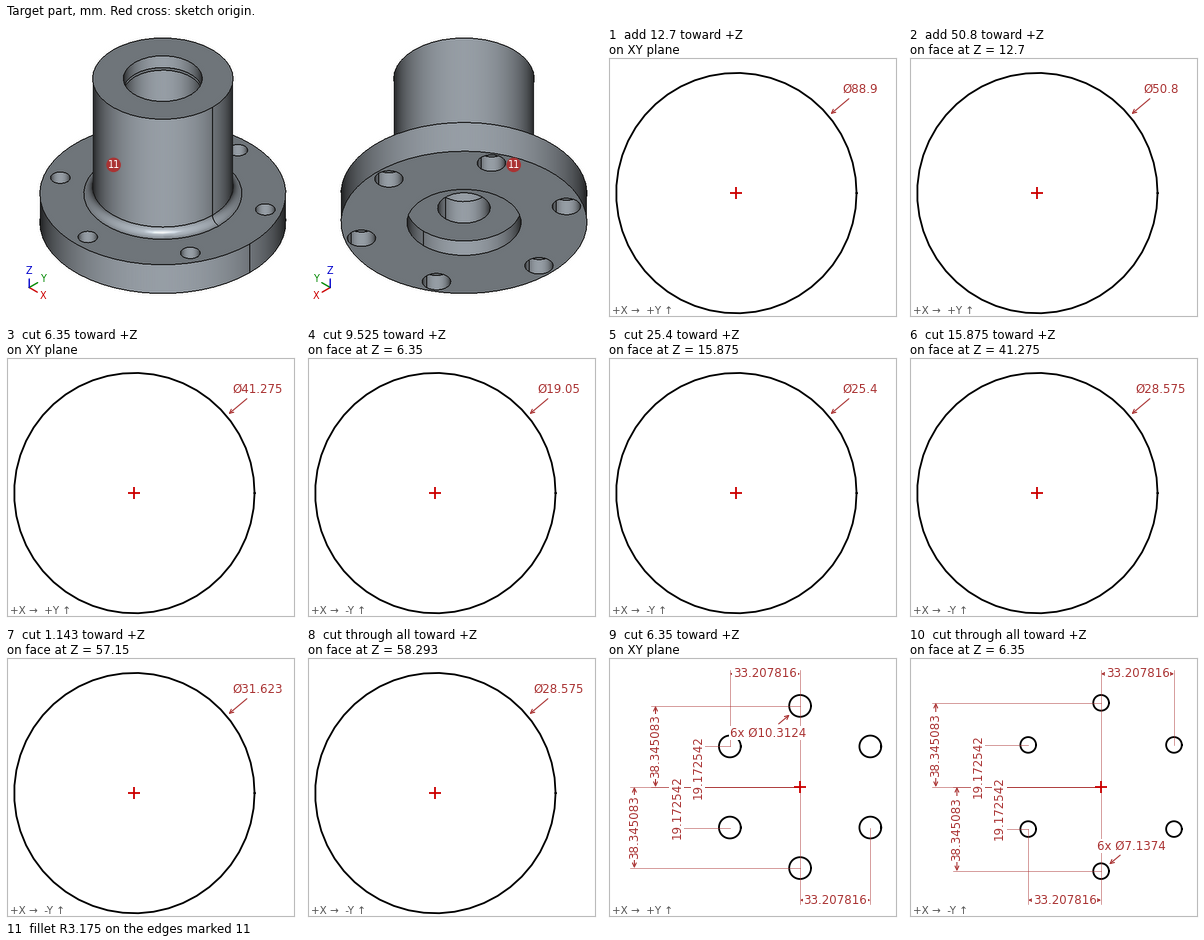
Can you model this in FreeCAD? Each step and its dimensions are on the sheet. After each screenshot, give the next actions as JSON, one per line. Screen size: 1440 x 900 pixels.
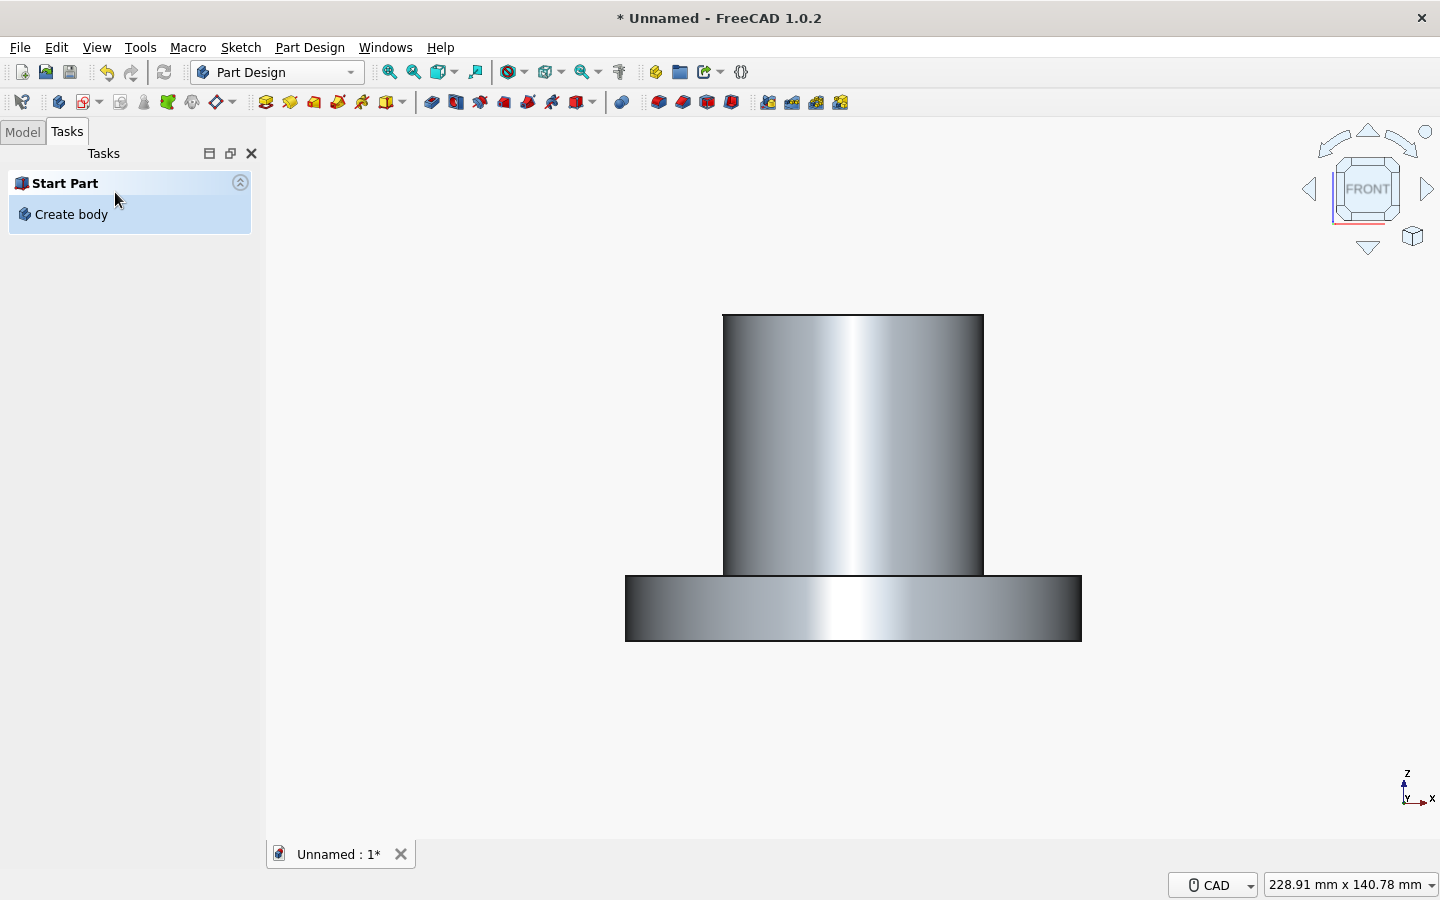
{"action": "key", "text": "3"}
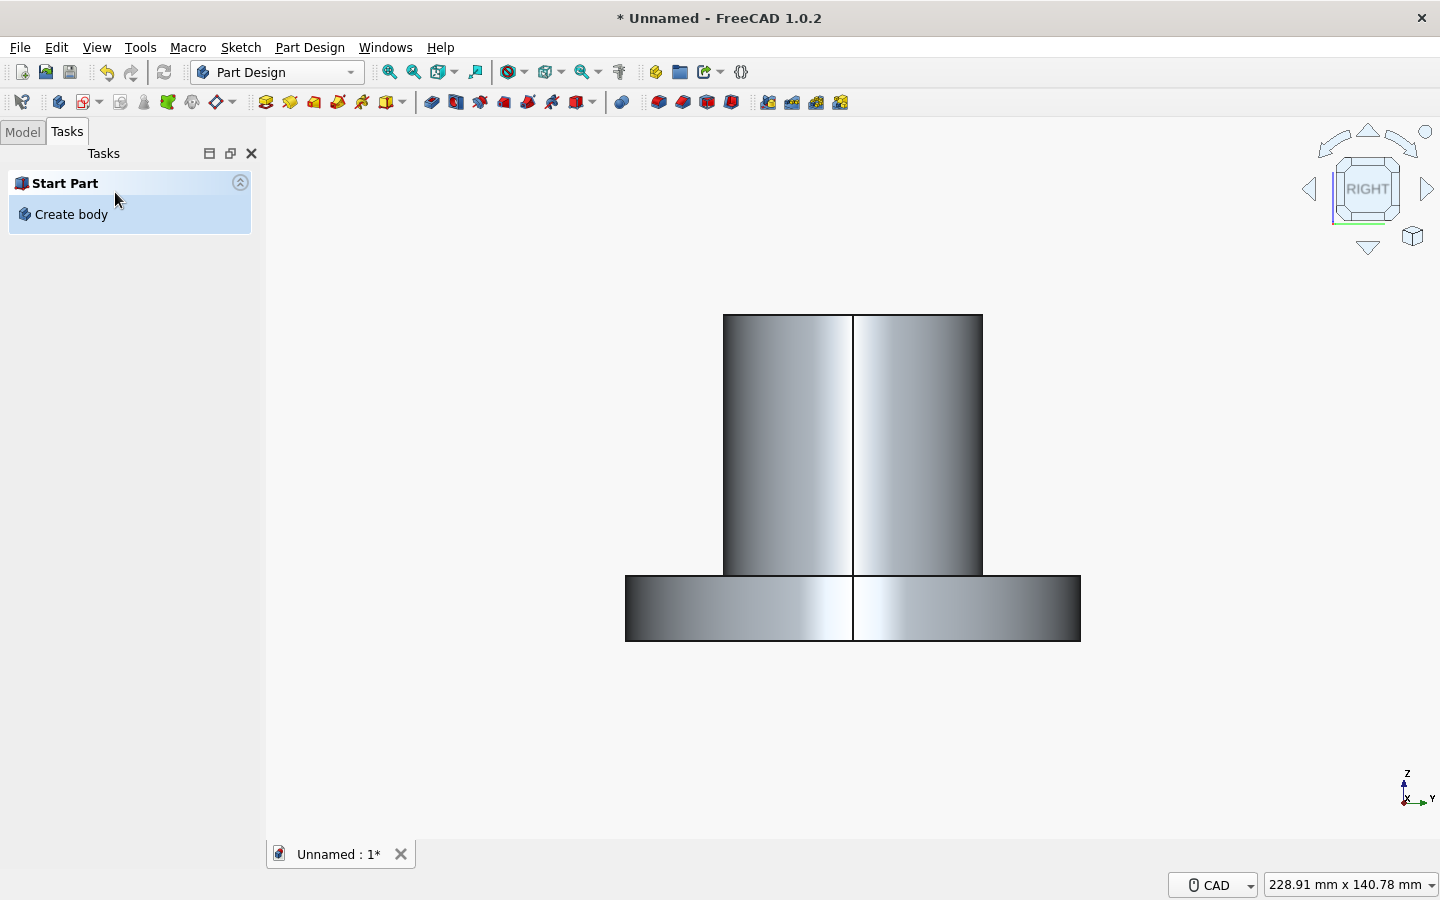
{"action": "key", "text": "5"}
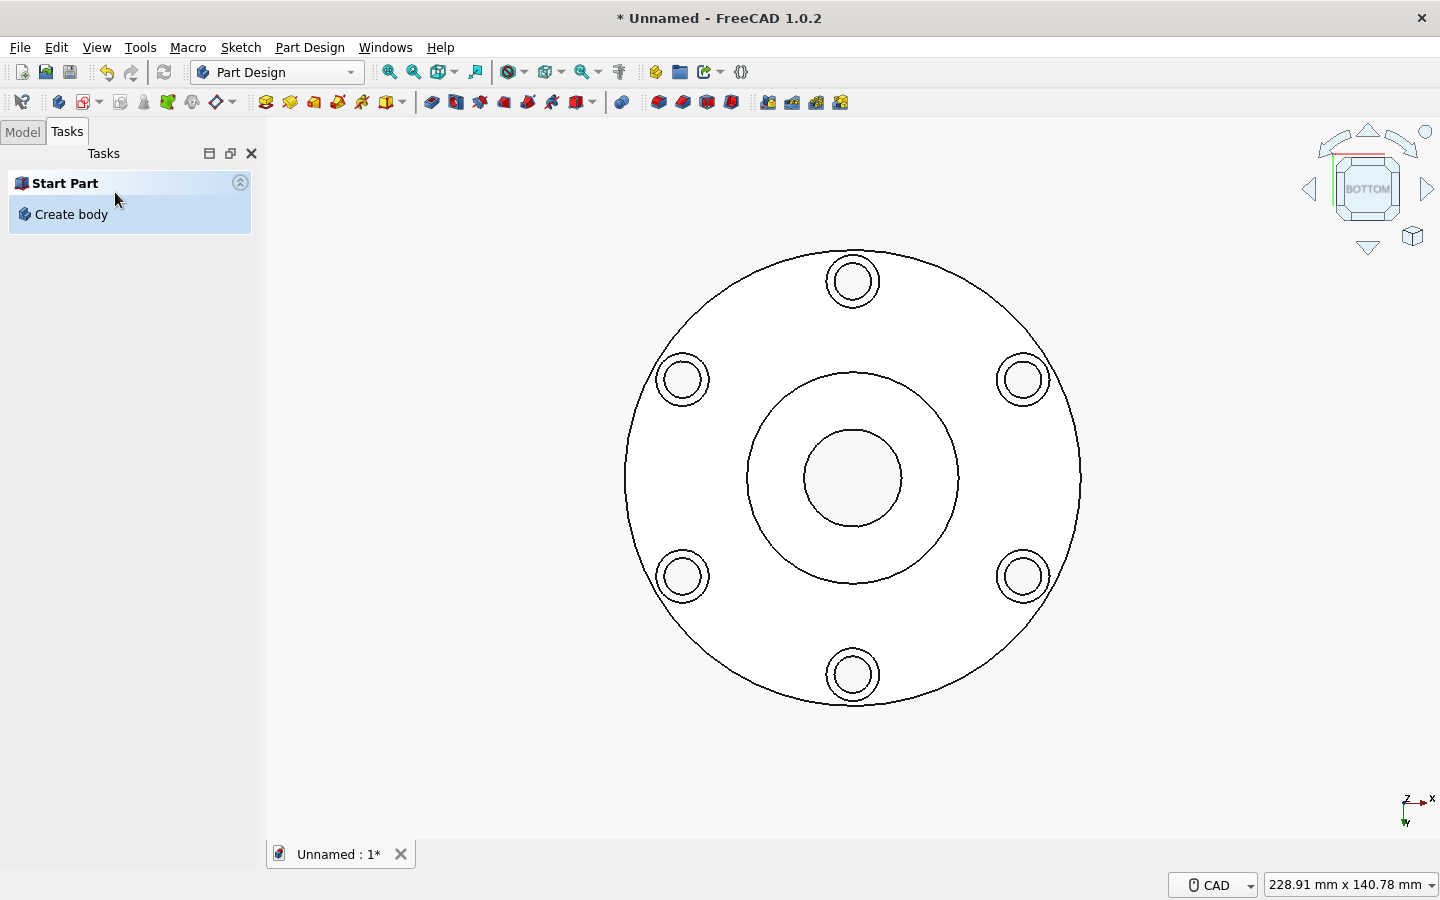
{"action": "key", "text": "4"}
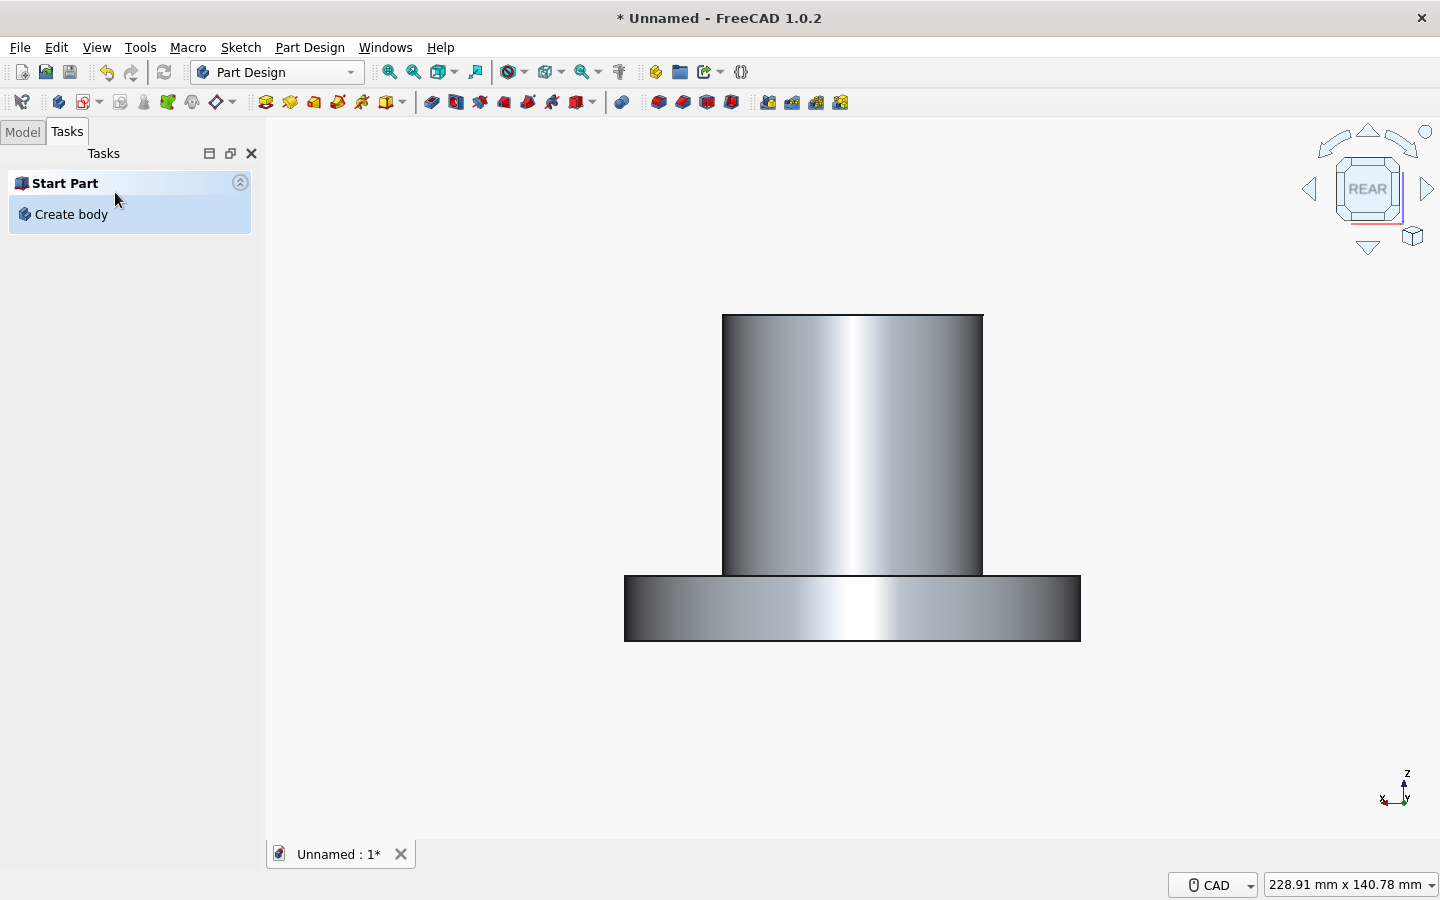
{"action": "key", "text": "6"}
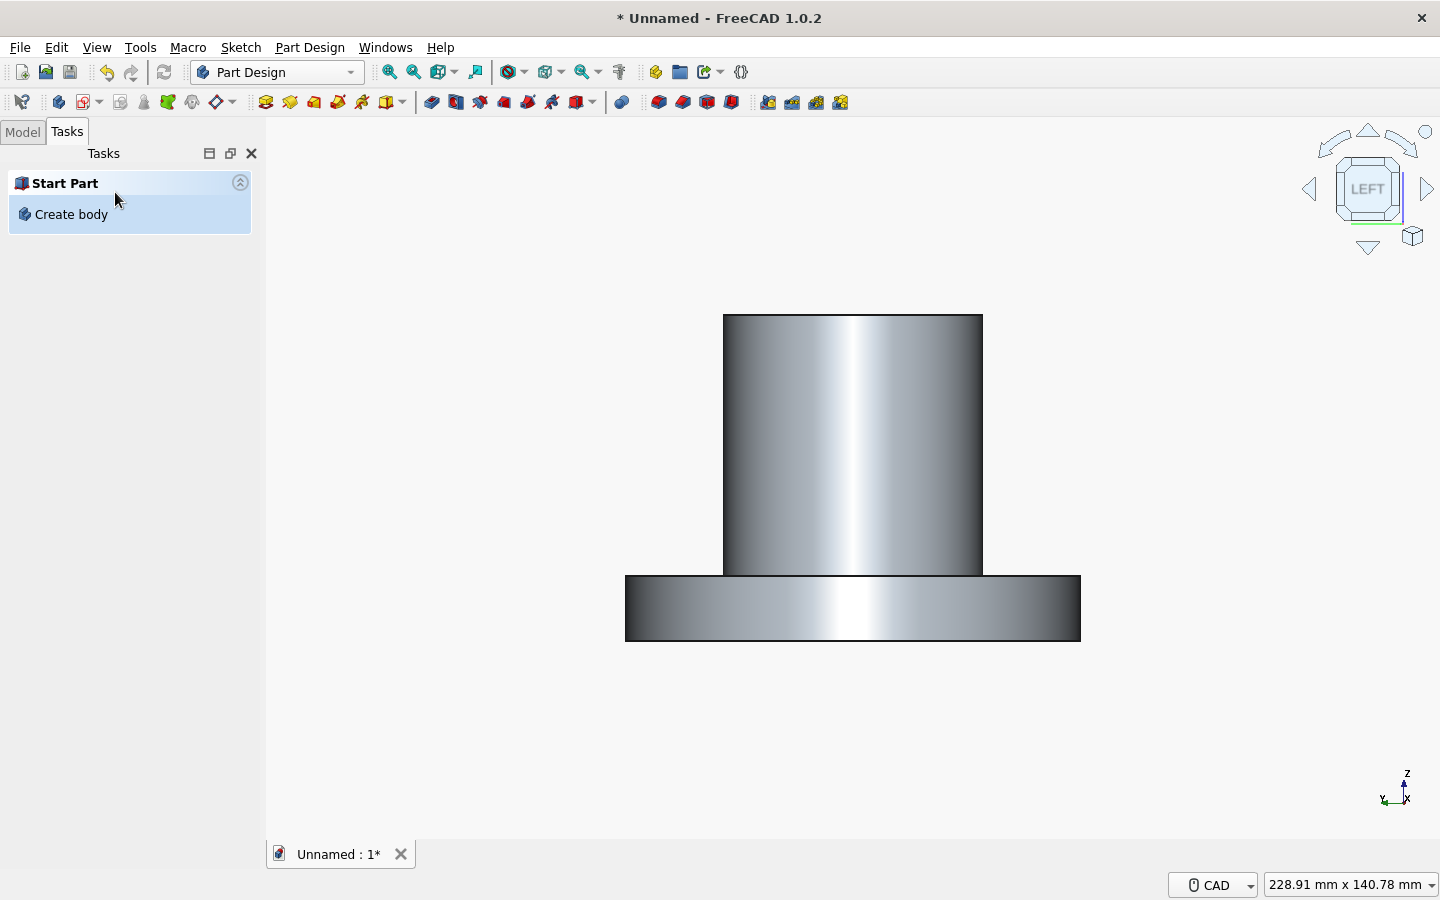
{"action": "key", "text": "v 3"}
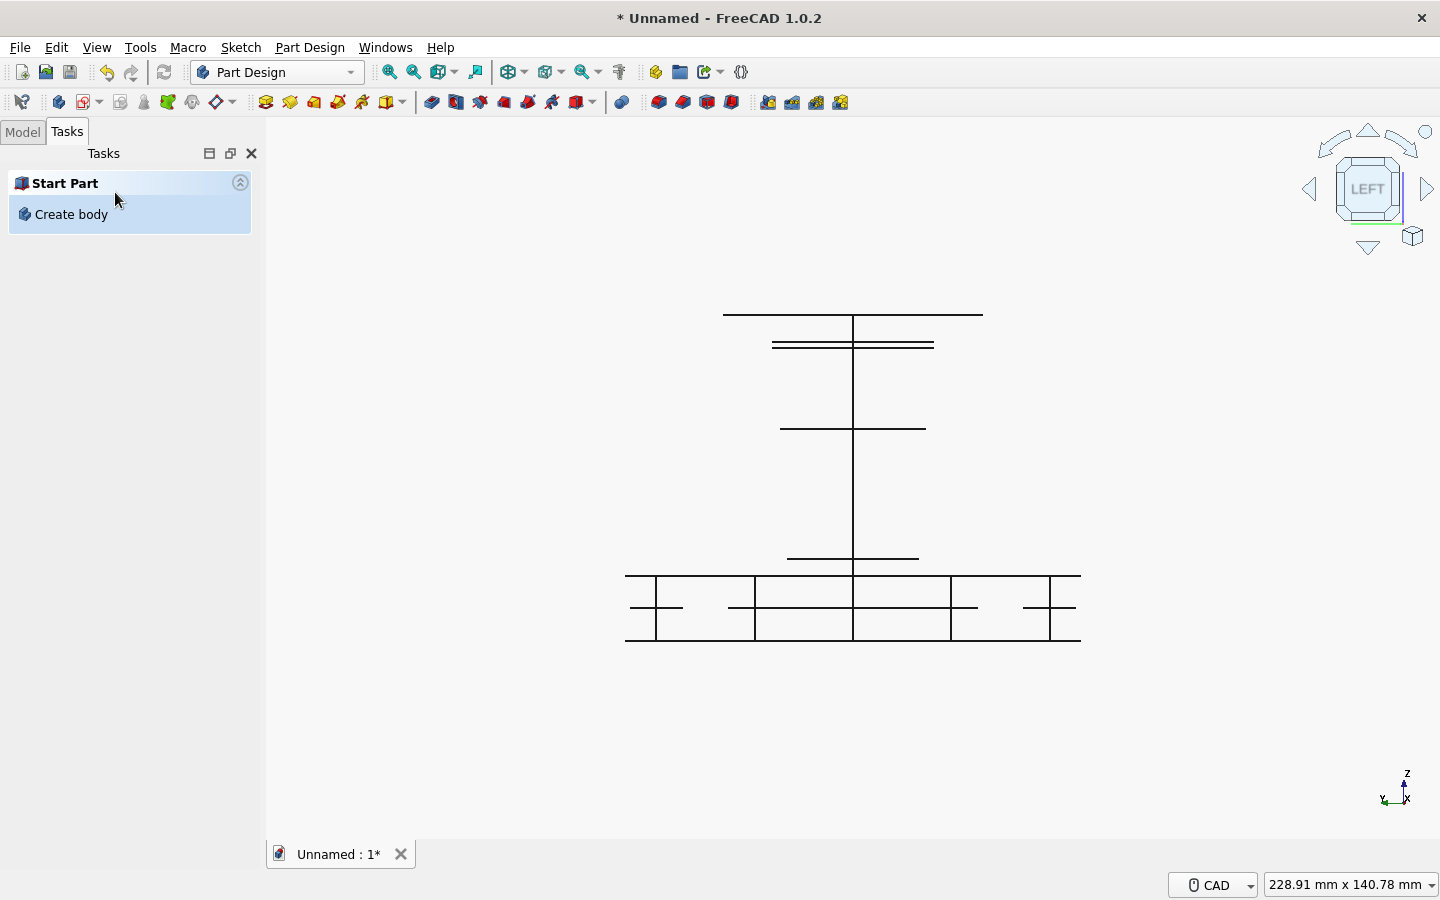
{"action": "key", "text": "0"}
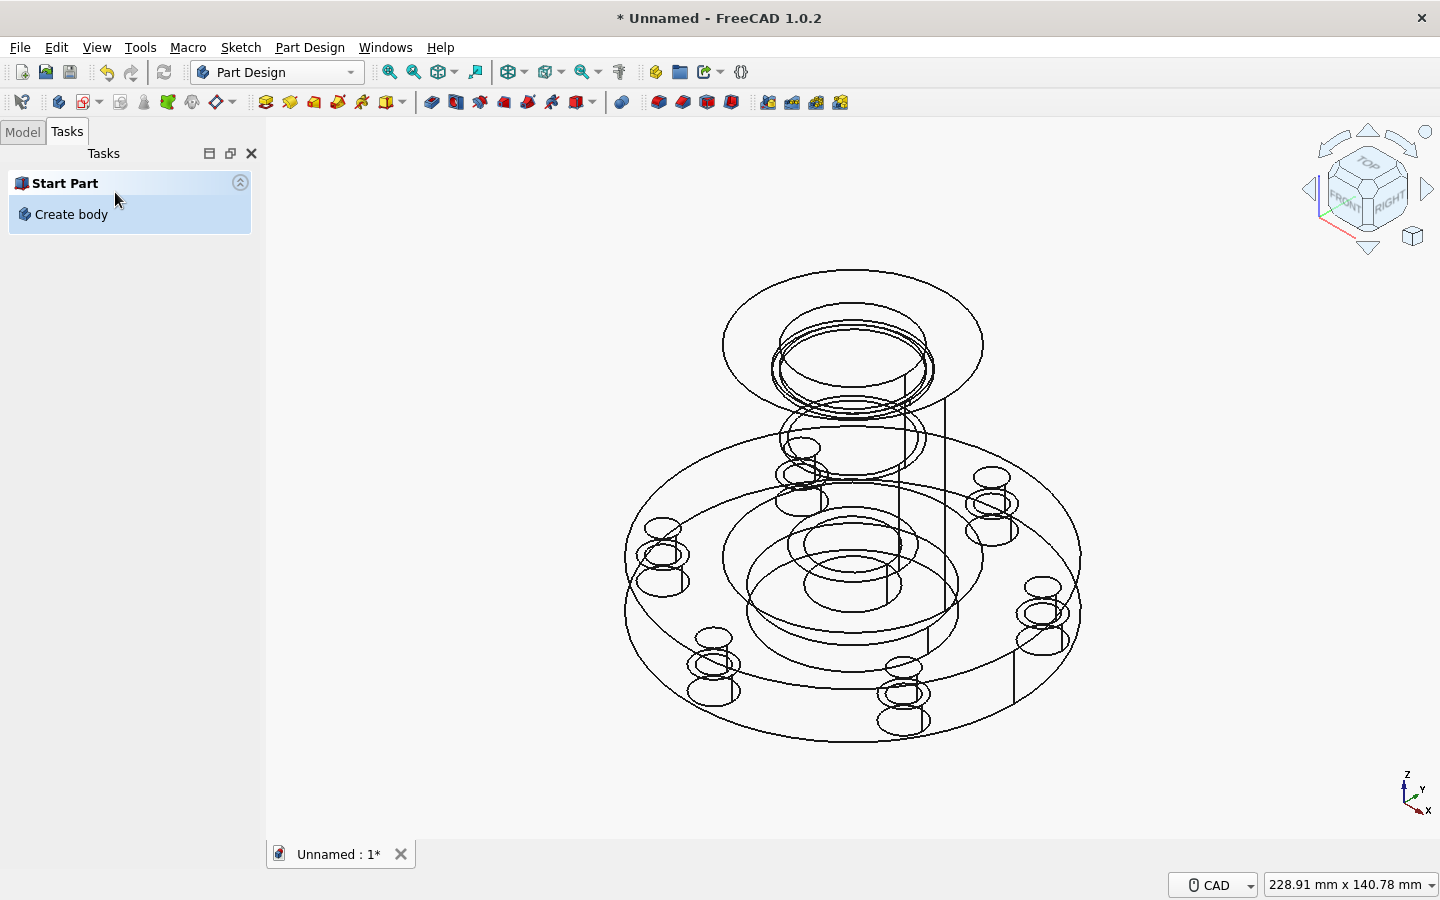
{"action": "left_click", "coordinate": [761, 504]}